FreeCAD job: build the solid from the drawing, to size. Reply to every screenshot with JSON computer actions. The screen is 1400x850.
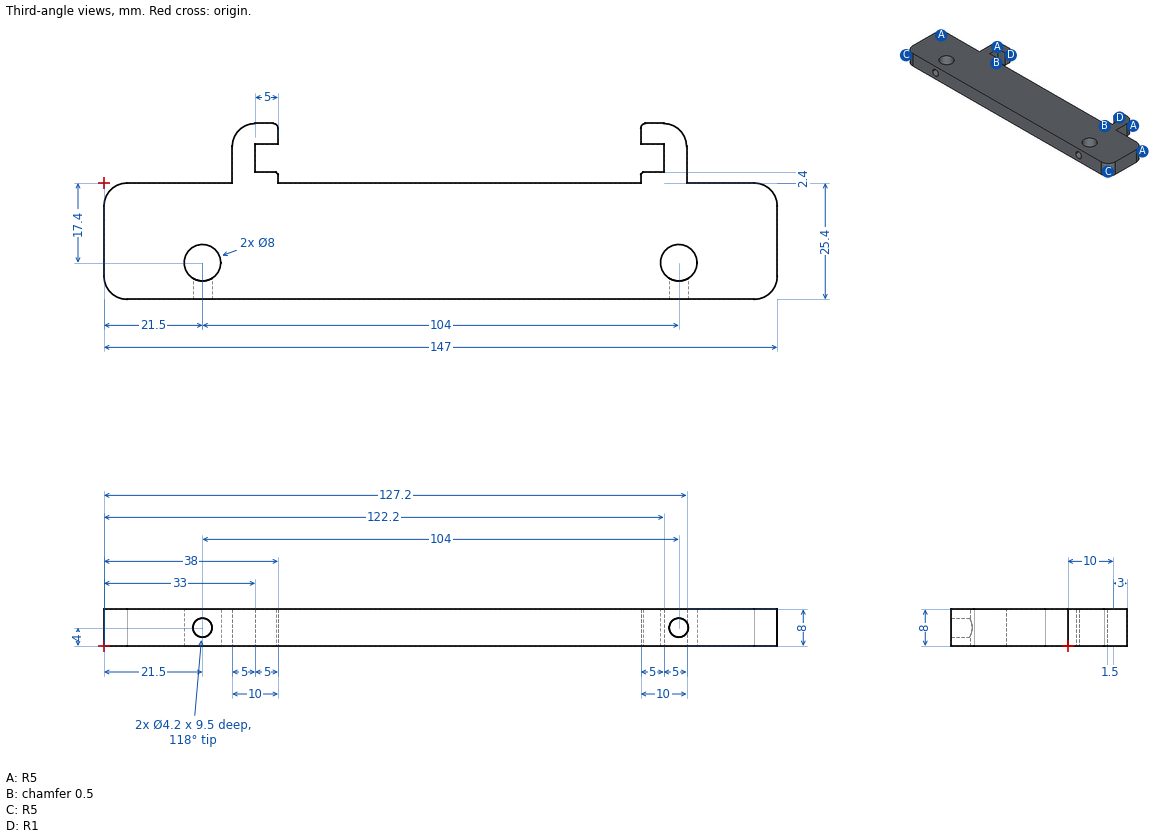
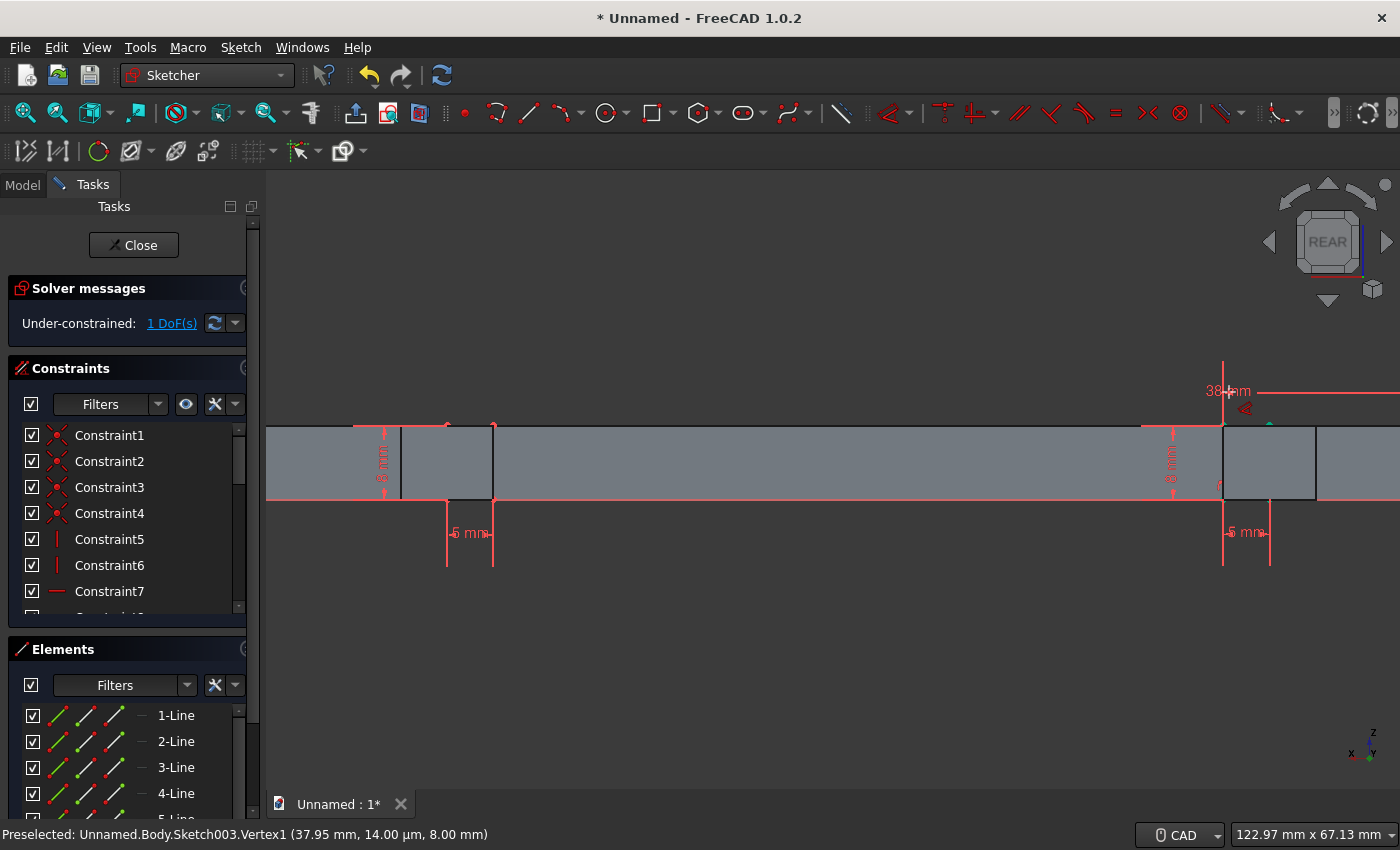
{"action": "left_click", "coordinate": [447, 426]}
{"action": "left_click", "coordinate": [841, 534]}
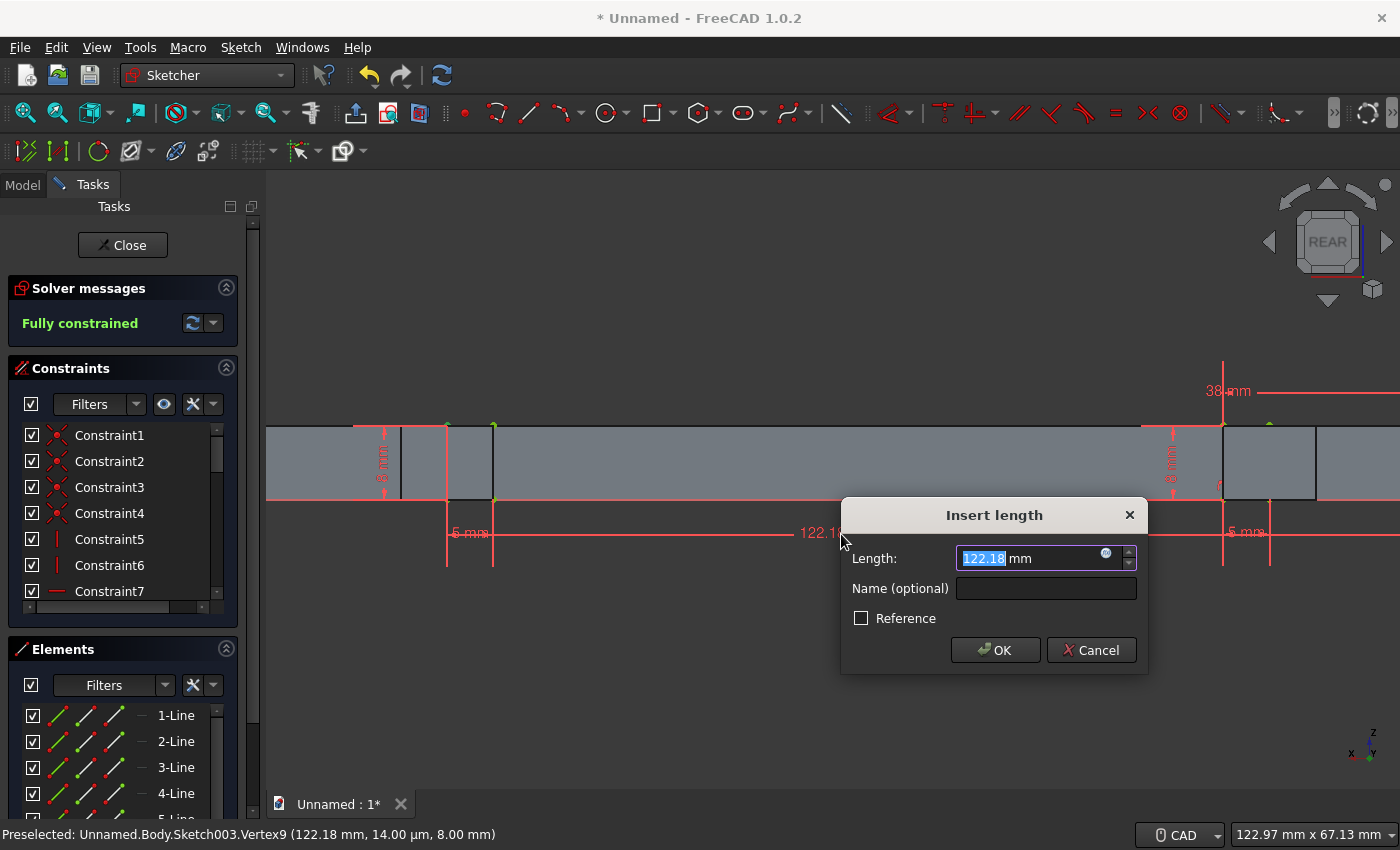
{"action": "type", "text": "122.2"}
{"action": "key", "text": "Return"}
{"action": "key", "text": "Escape"}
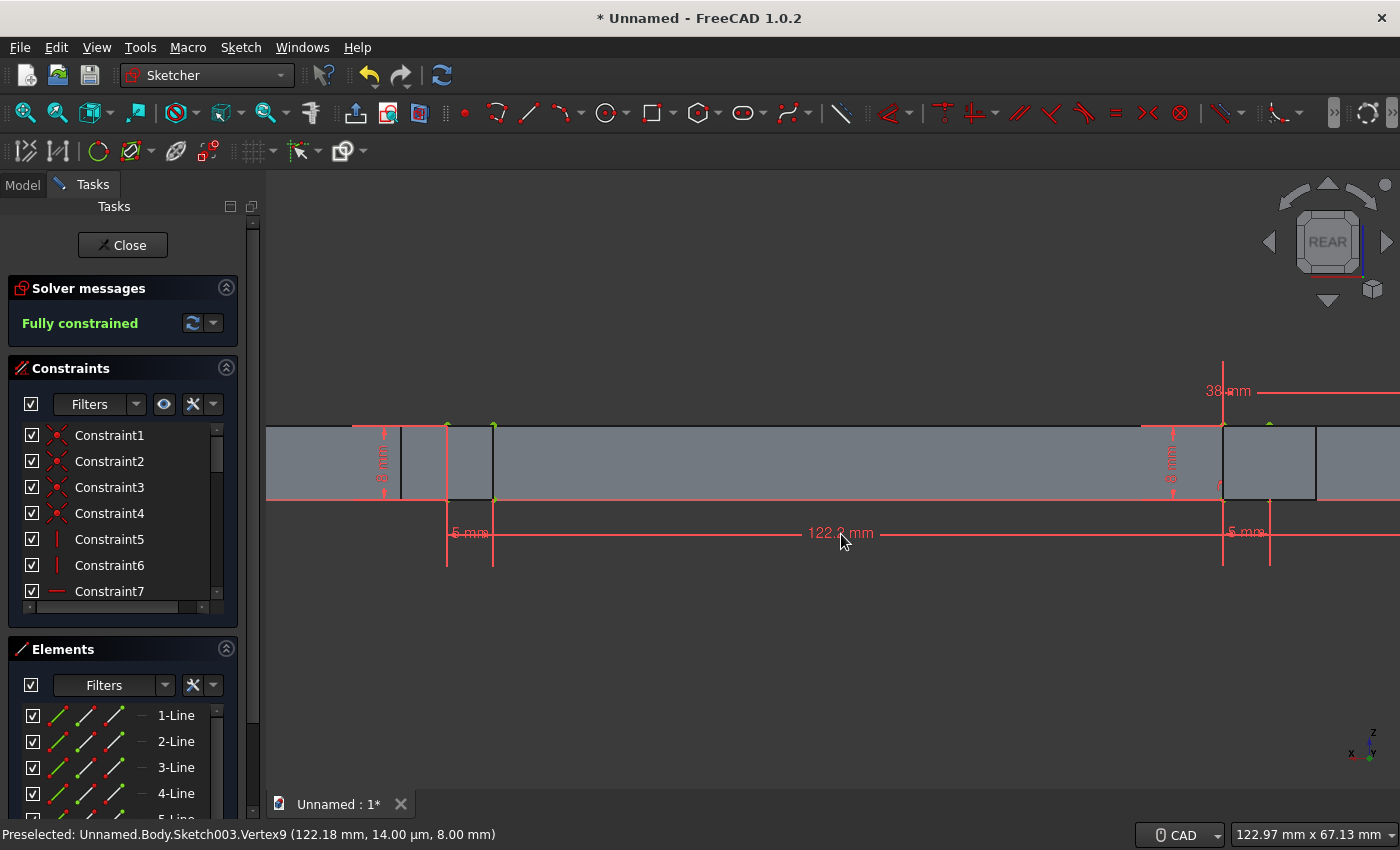
{"action": "left_click", "coordinate": [123, 245]}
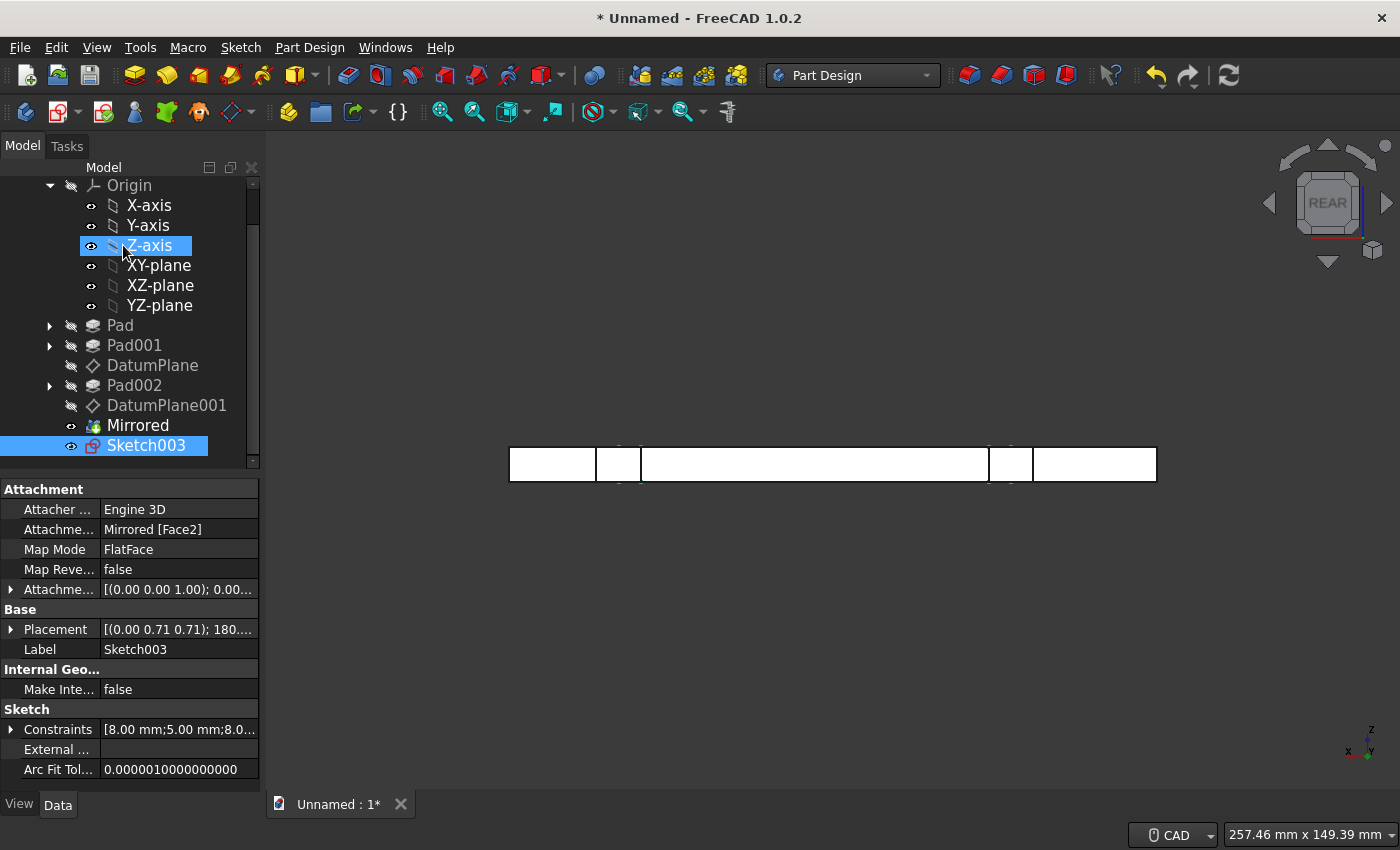
{"action": "left_click", "coordinate": [136, 76]}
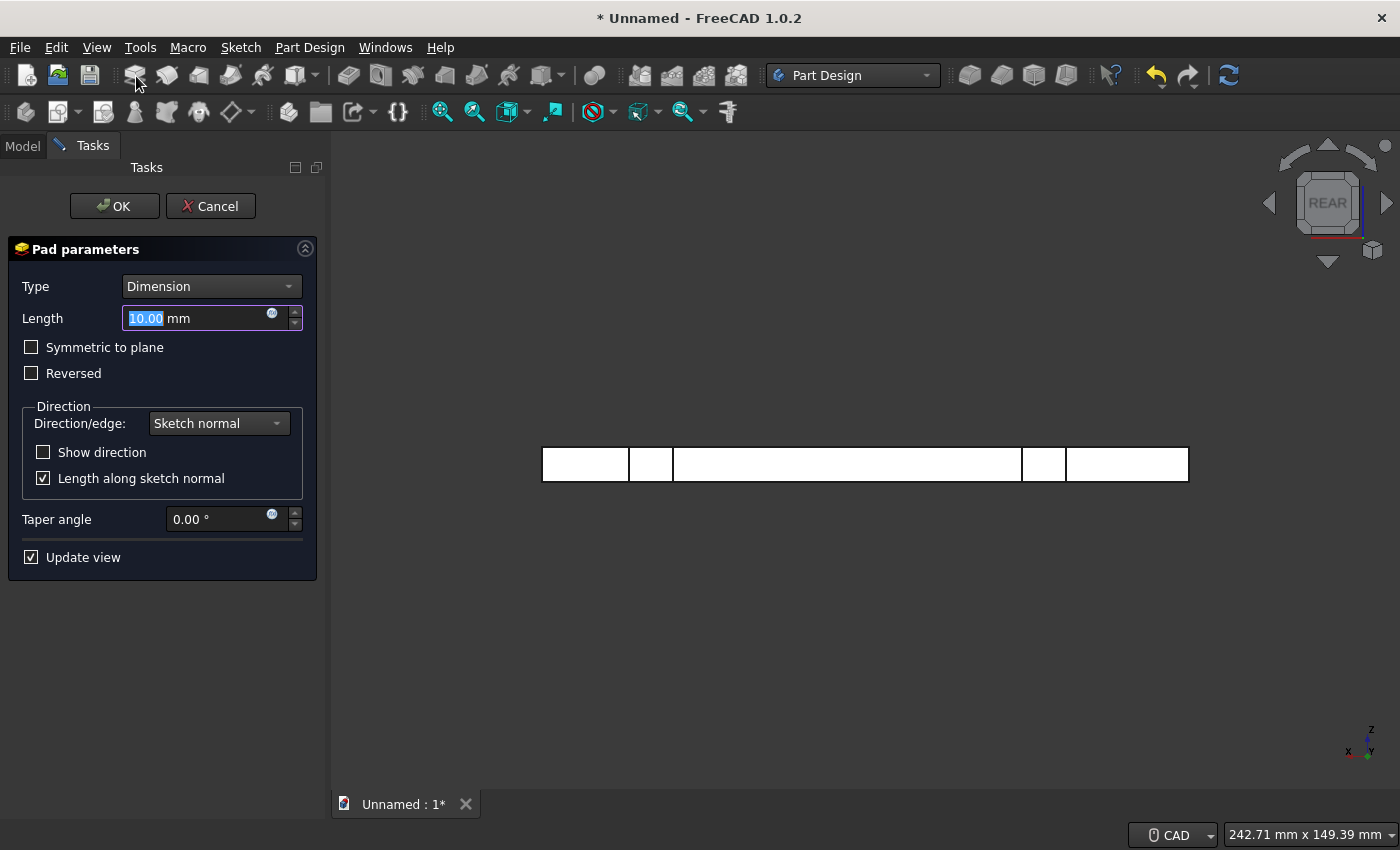
{"action": "type", "text": "2.4"}
{"action": "key", "text": "Tab"}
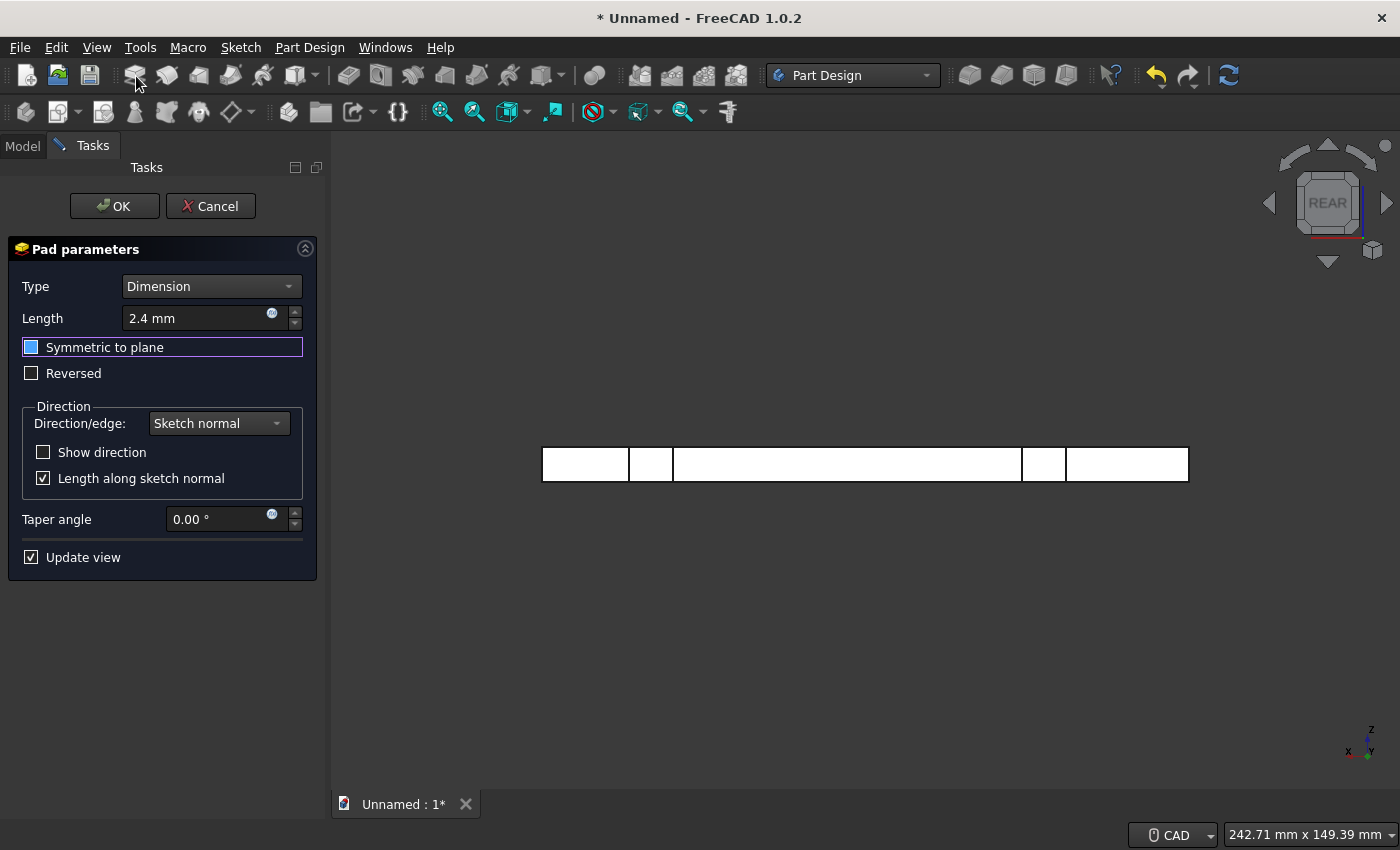
{"action": "left_click", "coordinate": [115, 206]}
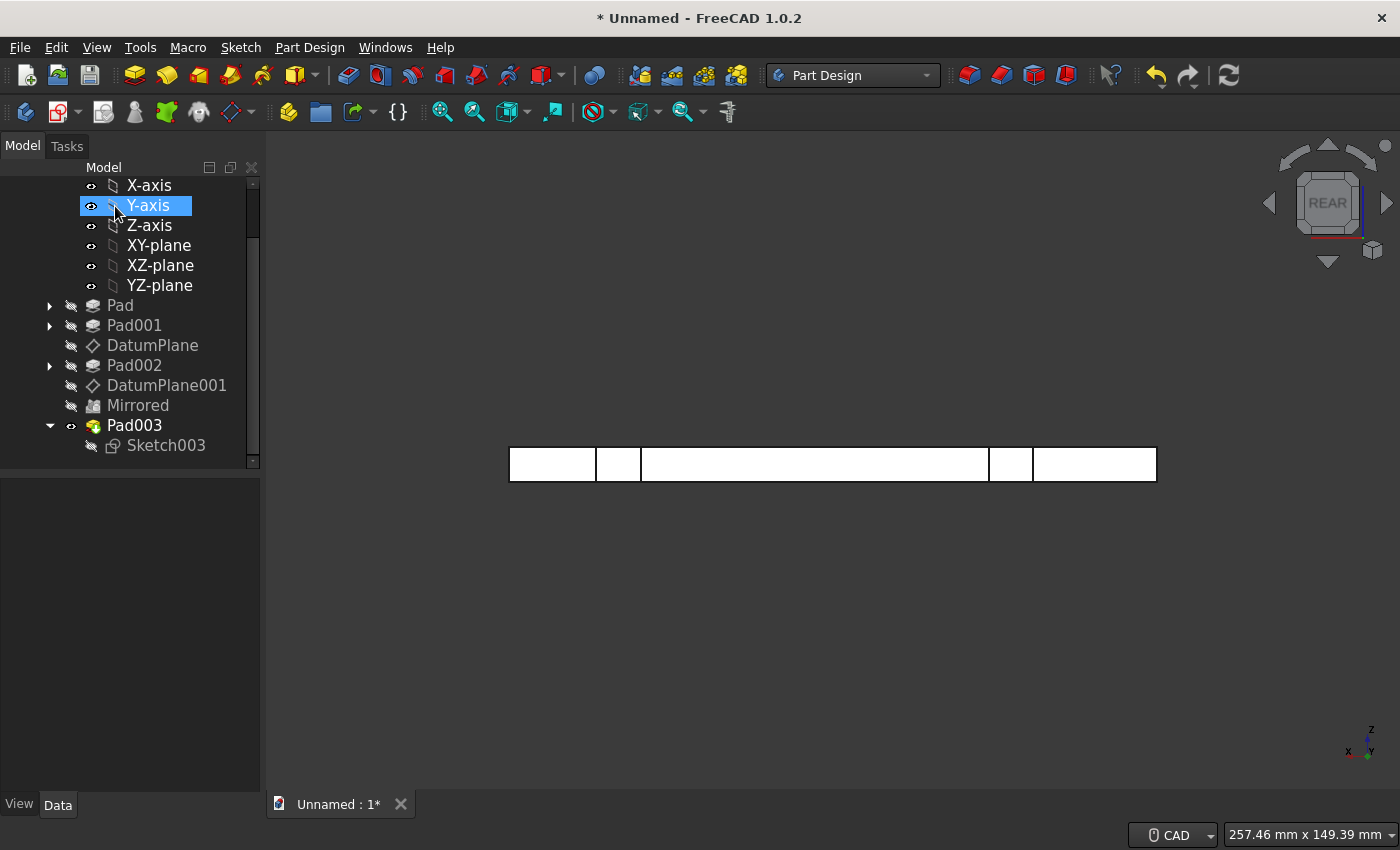
{"action": "key", "text": "0"}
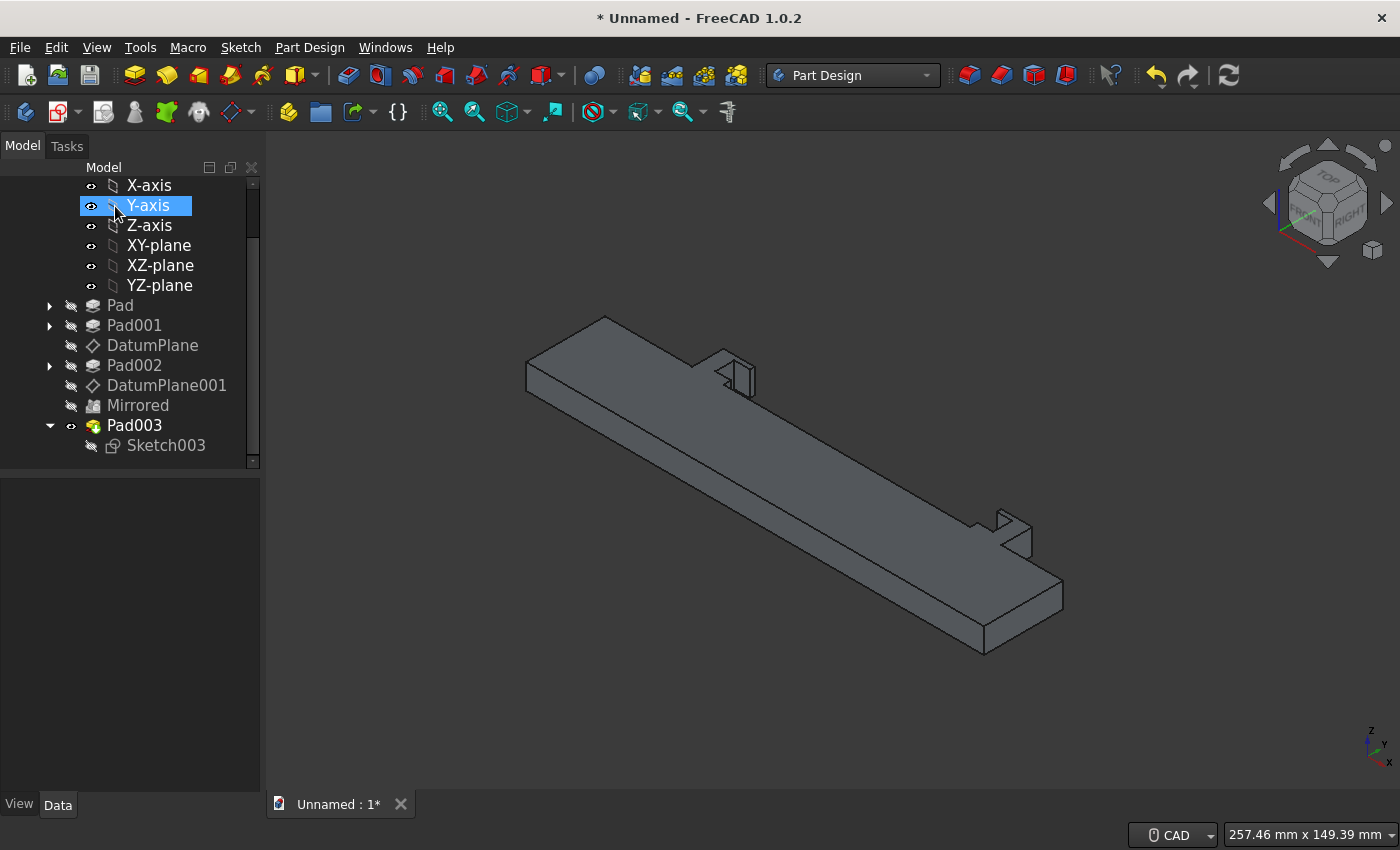
{"action": "left_click", "coordinate": [925, 546]}